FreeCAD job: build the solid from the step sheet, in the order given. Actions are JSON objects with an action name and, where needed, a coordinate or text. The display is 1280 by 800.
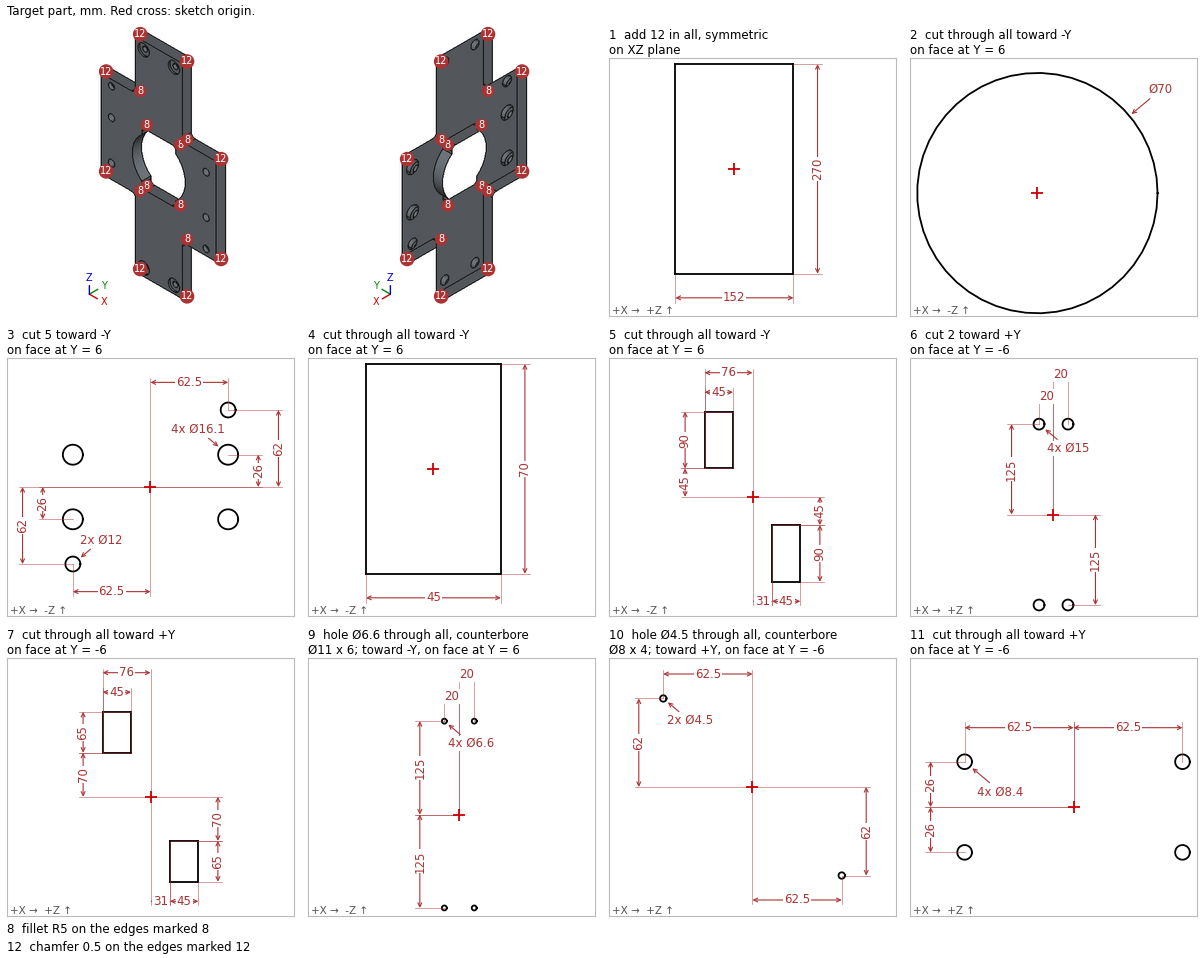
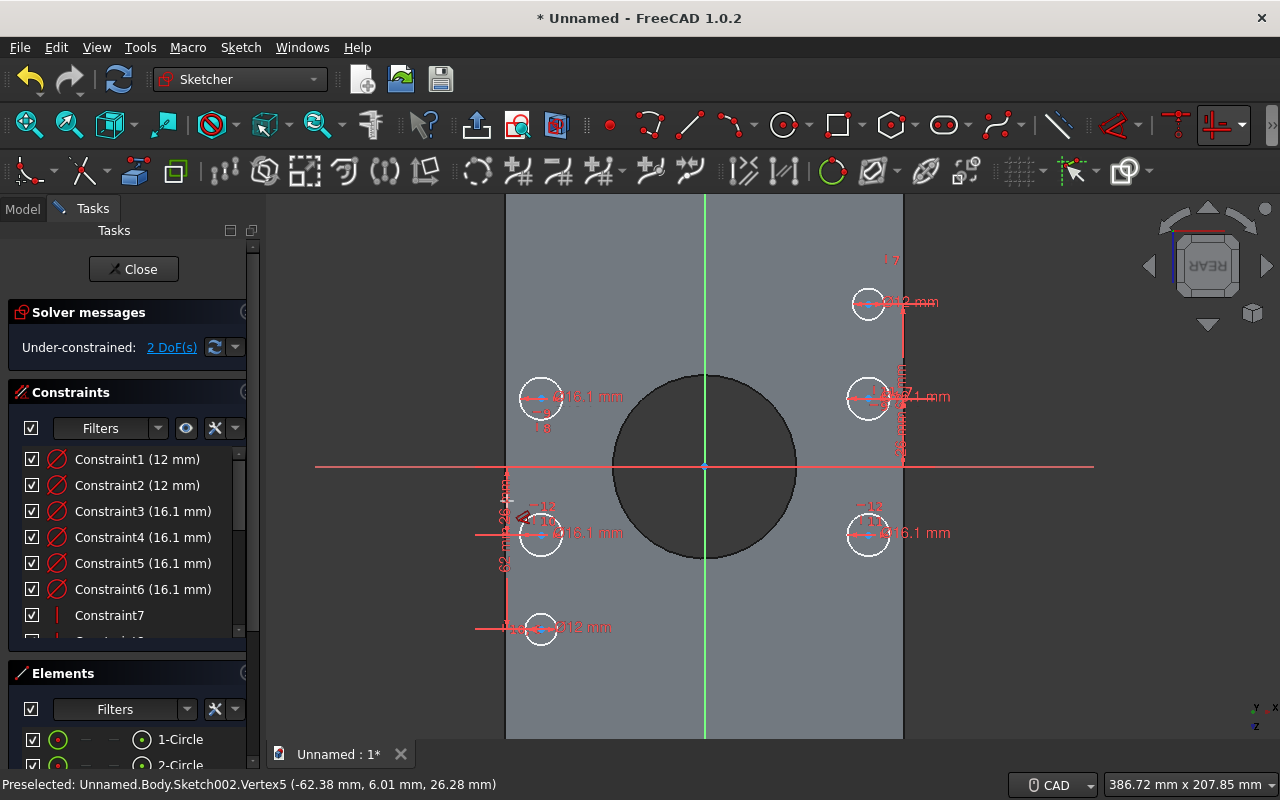
{"action": "left_click", "coordinate": [869, 304]}
{"action": "left_click", "coordinate": [787, 270]}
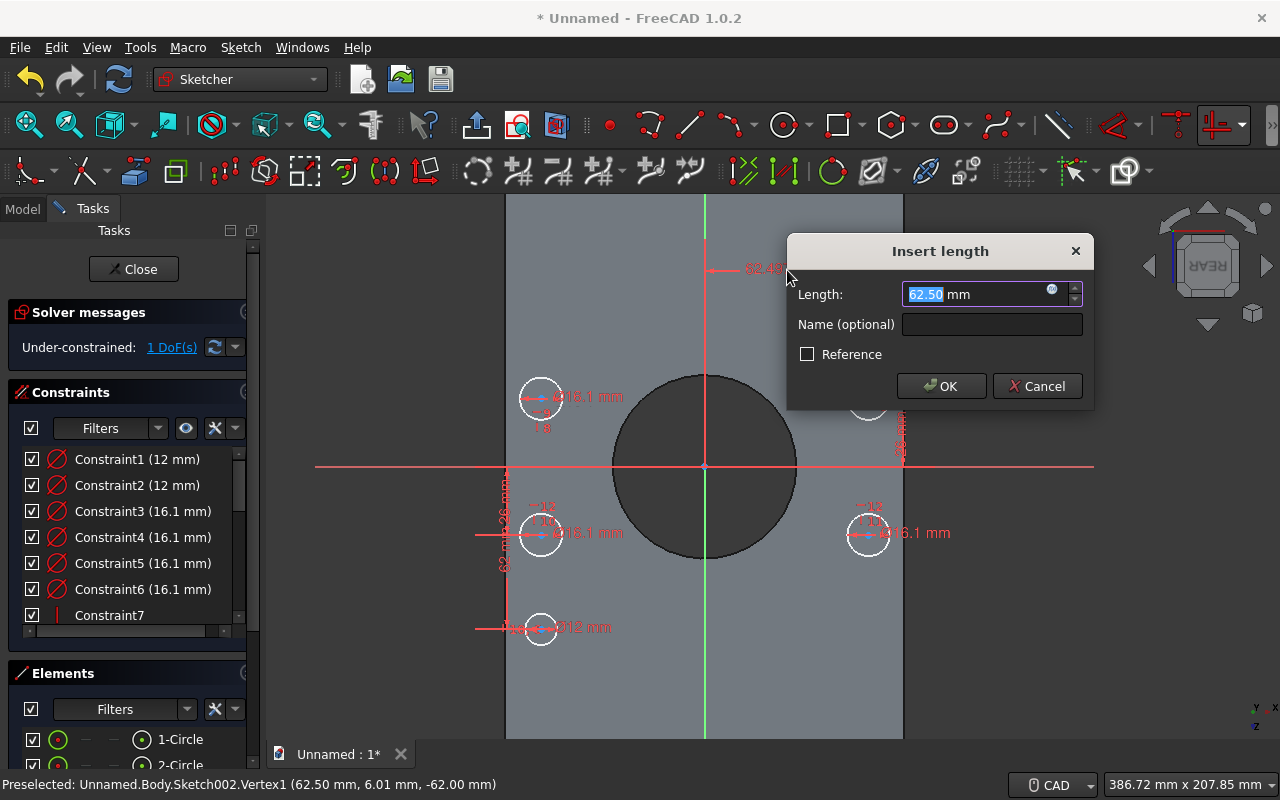
{"action": "type", "text": "62.5"}
{"action": "key", "text": "Return"}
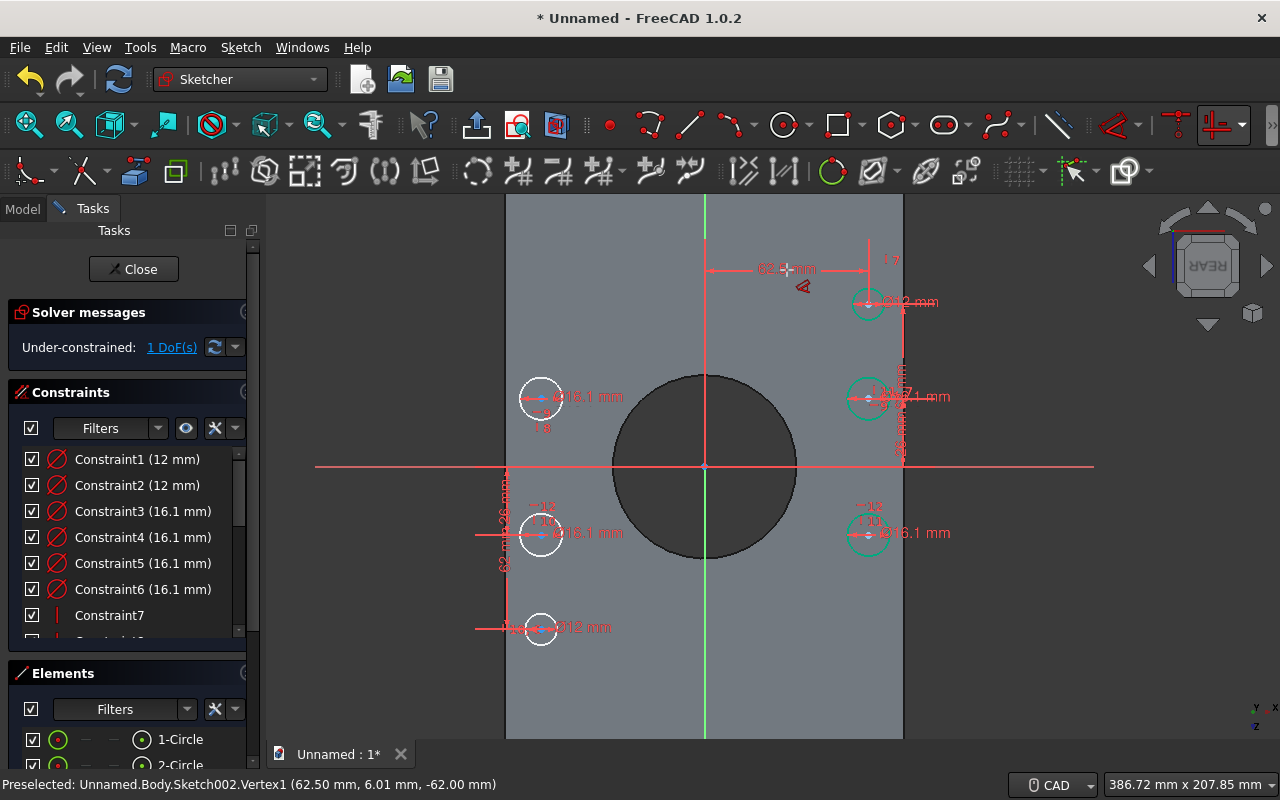
{"action": "left_click", "coordinate": [541, 629]}
{"action": "left_click", "coordinate": [623, 663]}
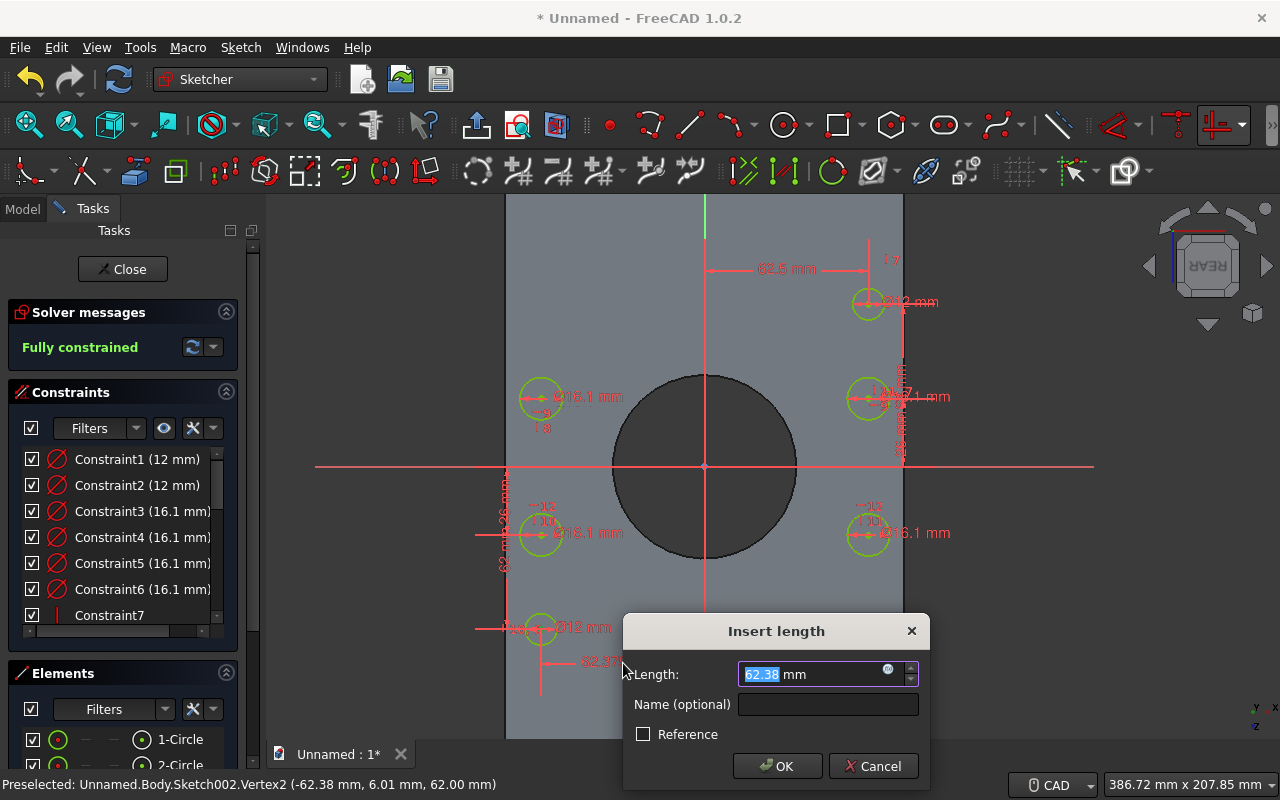
{"action": "type", "text": "62.5"}
{"action": "key", "text": "Return"}
{"action": "key", "text": "Escape"}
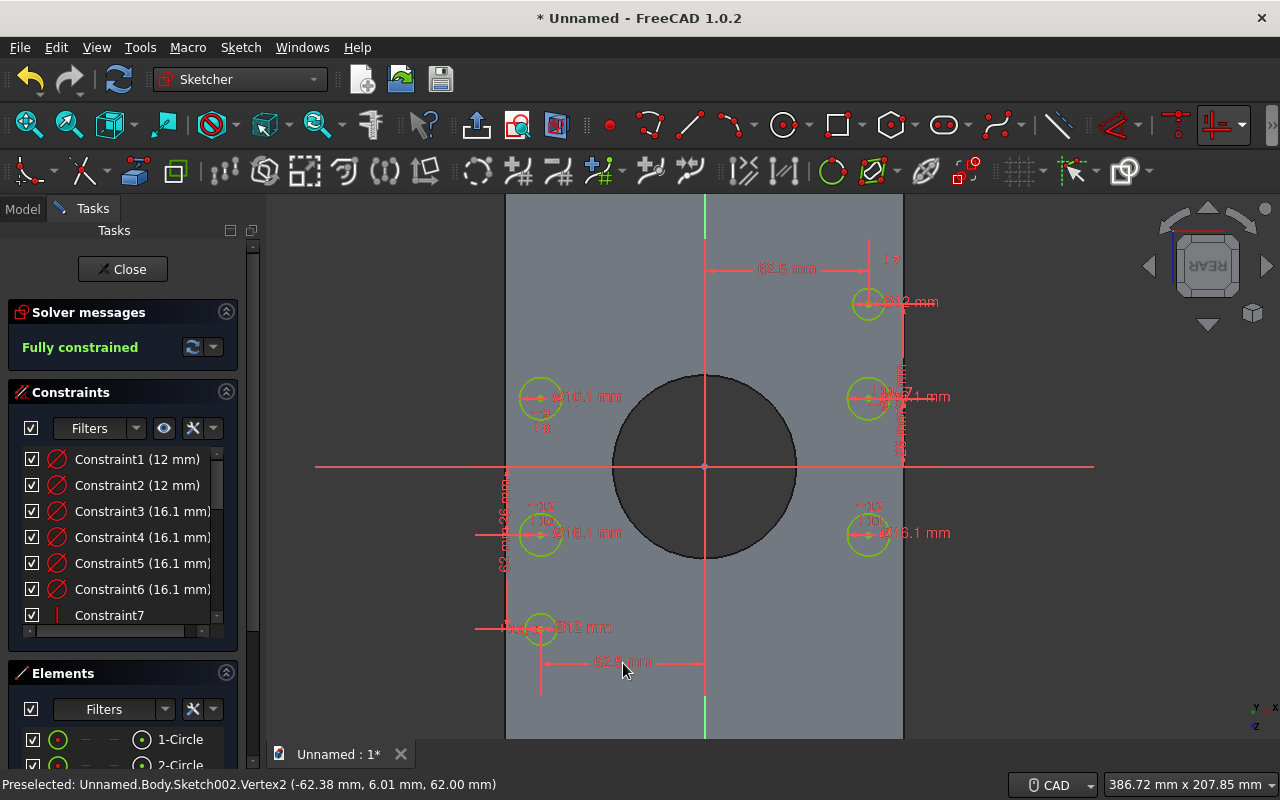
{"action": "left_click", "coordinate": [123, 269]}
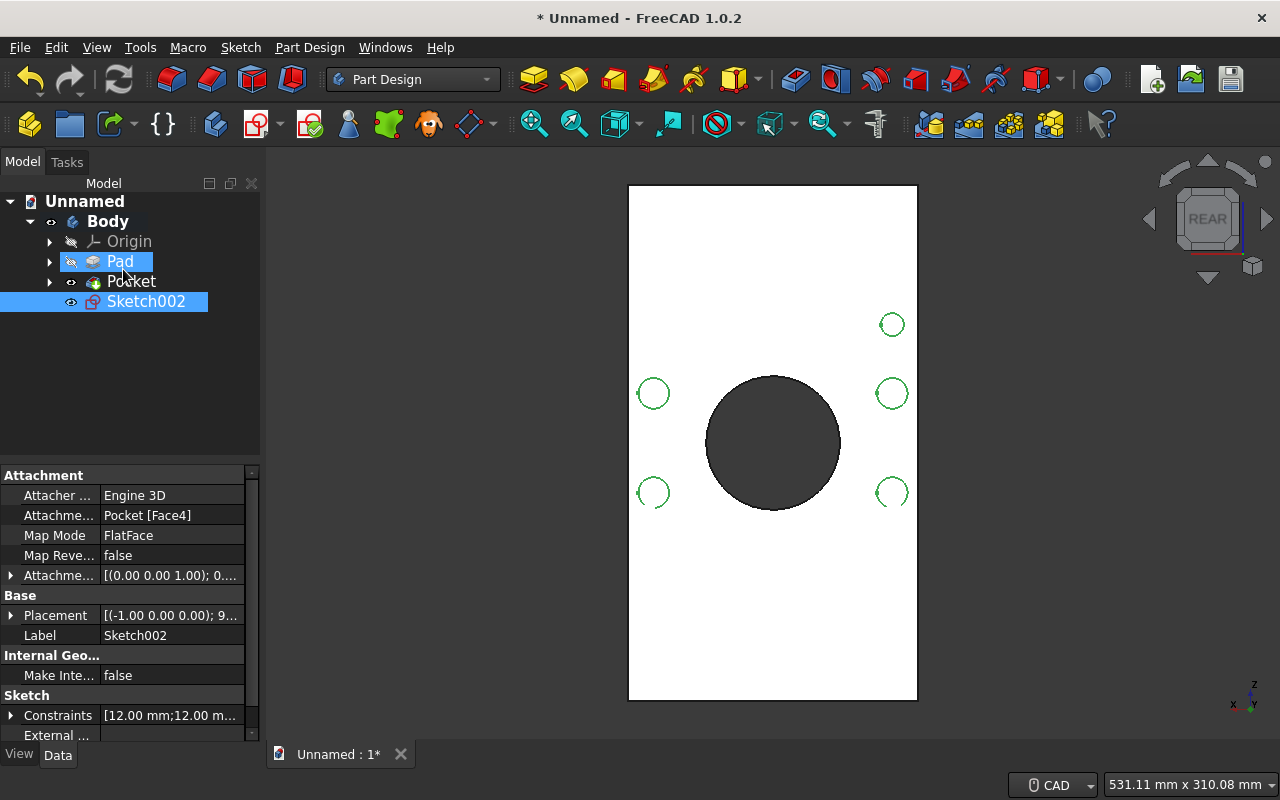
{"action": "left_click", "coordinate": [796, 80]}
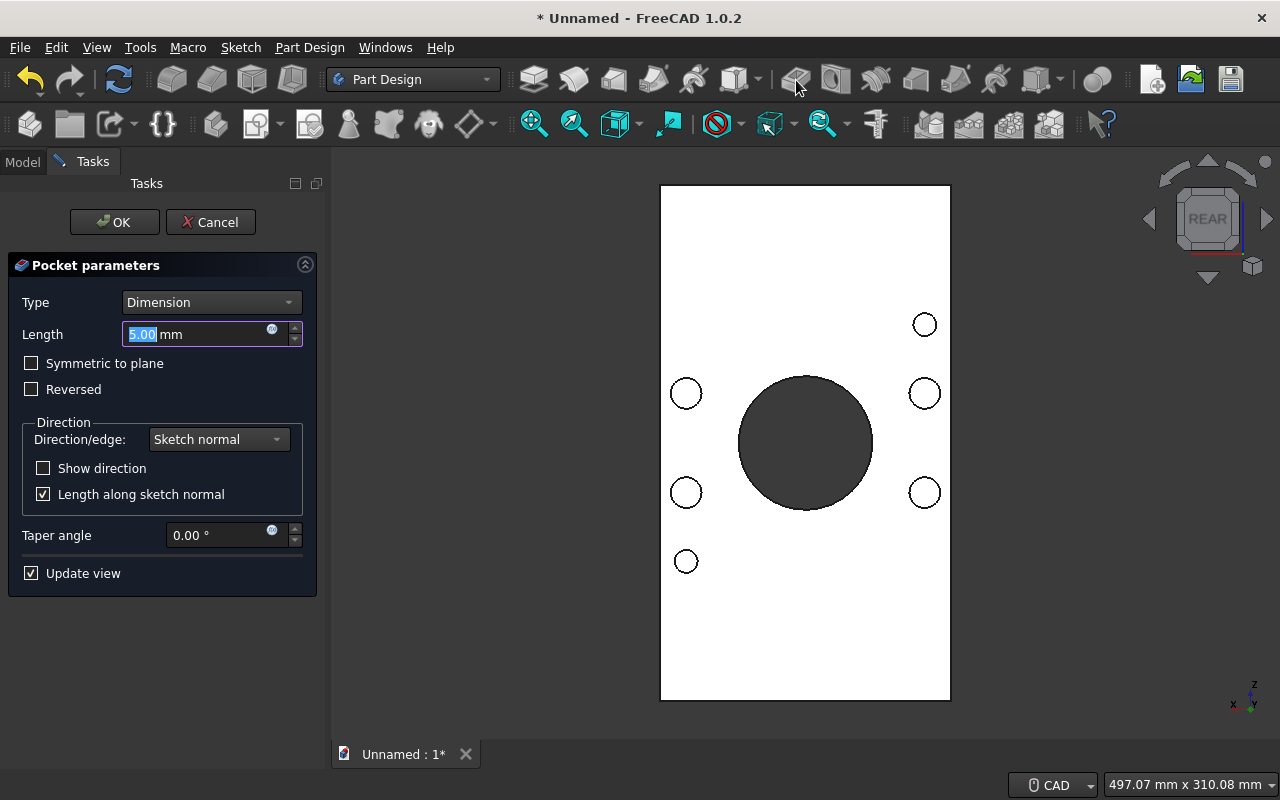
{"action": "type", "text": "5"}
{"action": "key", "text": "Tab"}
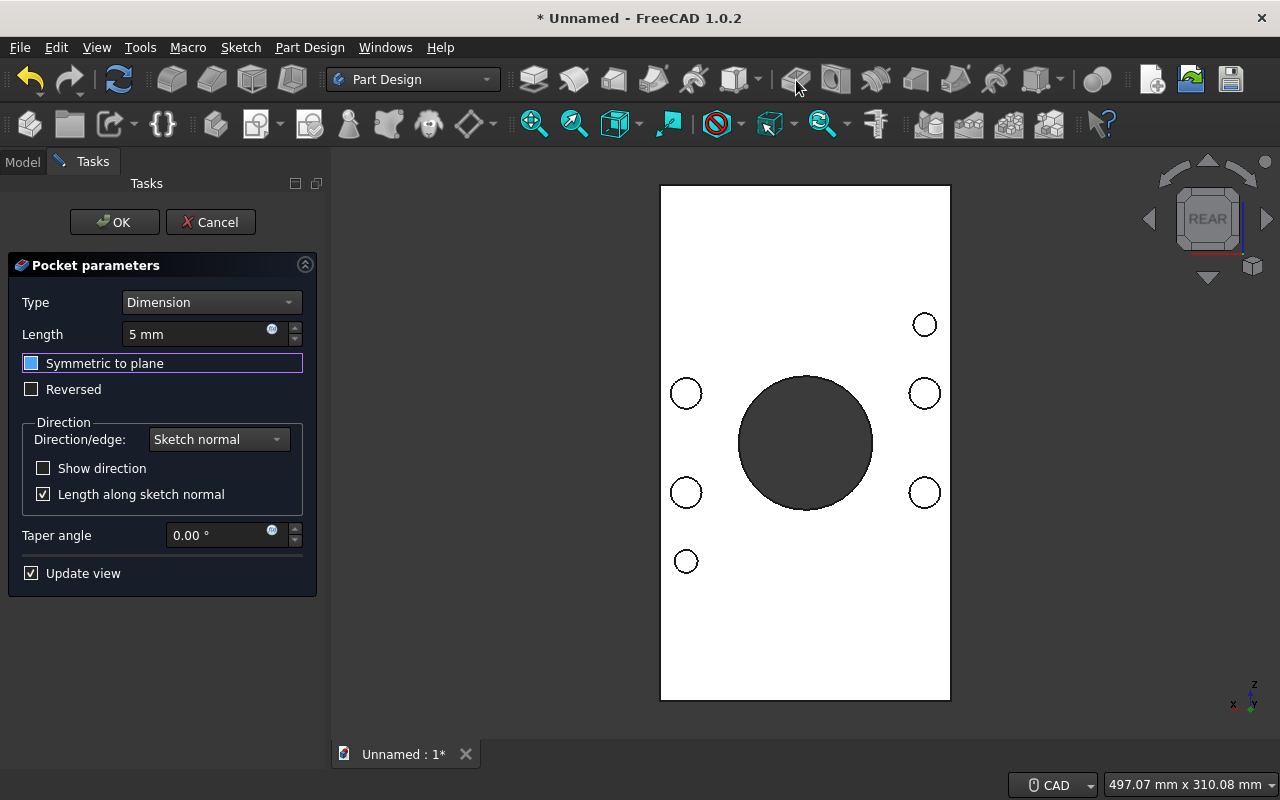
{"action": "left_click", "coordinate": [115, 222]}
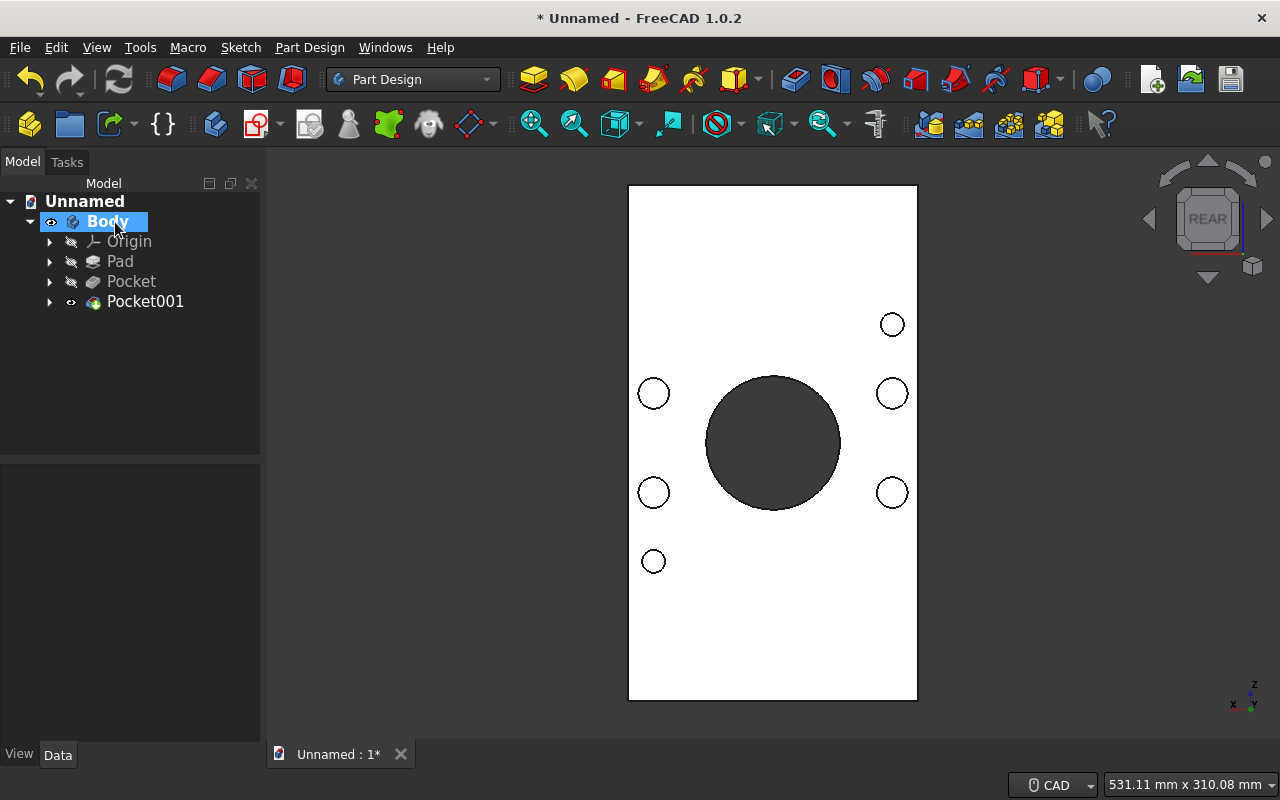
{"action": "left_click", "coordinate": [732, 295]}